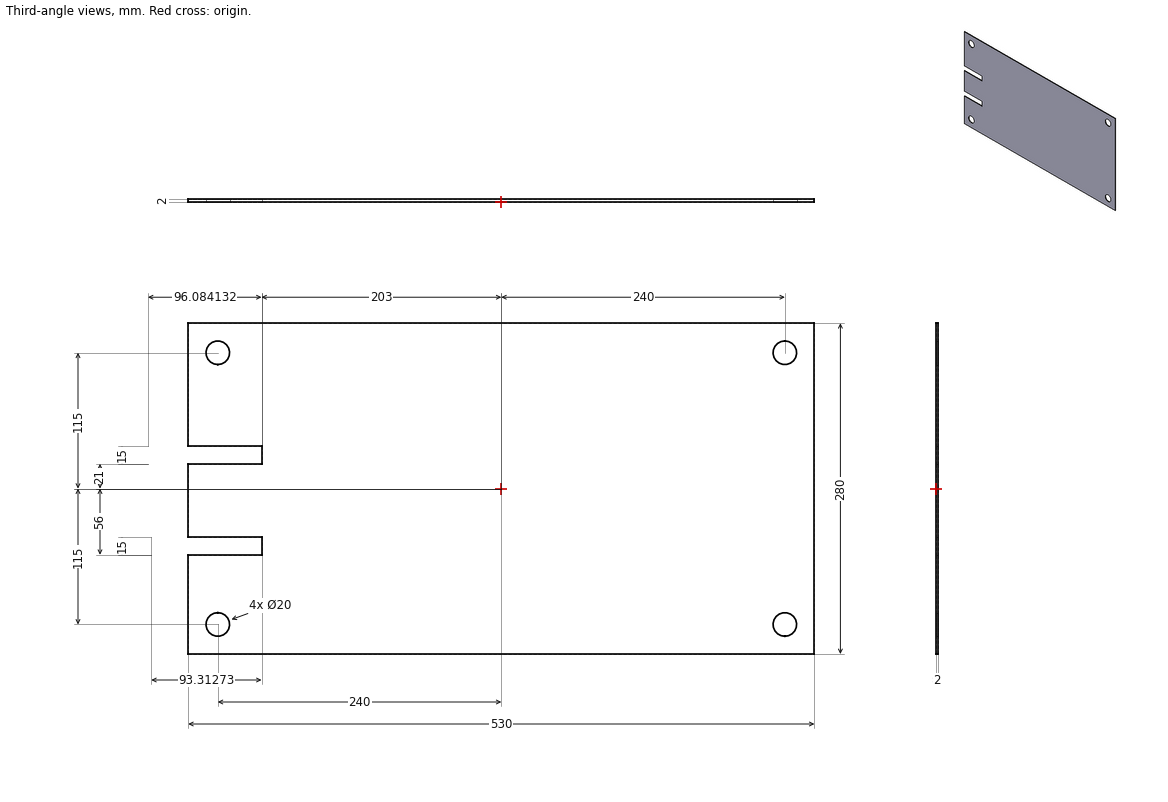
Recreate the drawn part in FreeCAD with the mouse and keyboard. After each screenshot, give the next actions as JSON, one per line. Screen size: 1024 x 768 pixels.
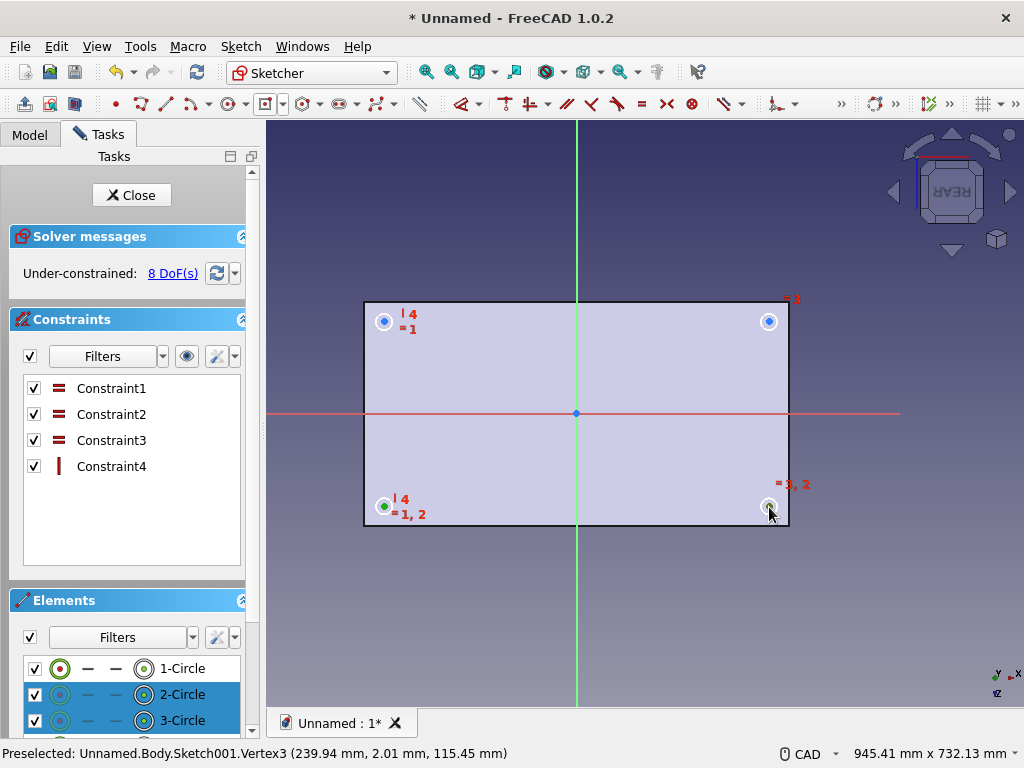
{"action": "left_click", "coordinate": [548, 104]}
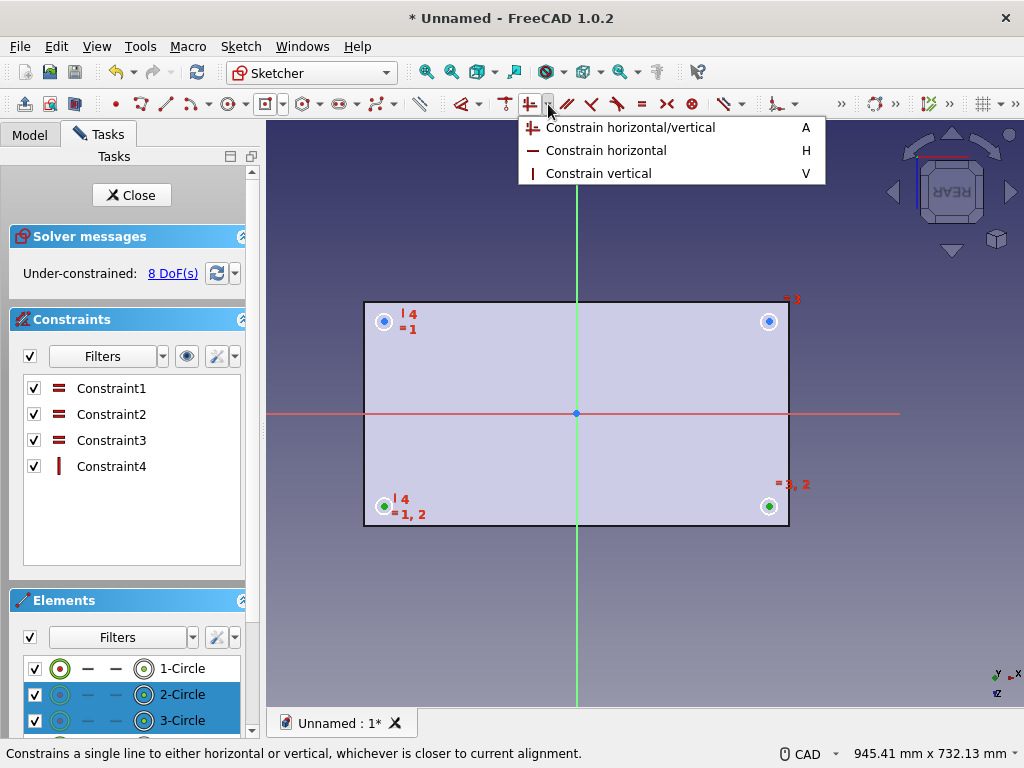
{"action": "left_click", "coordinate": [672, 150]}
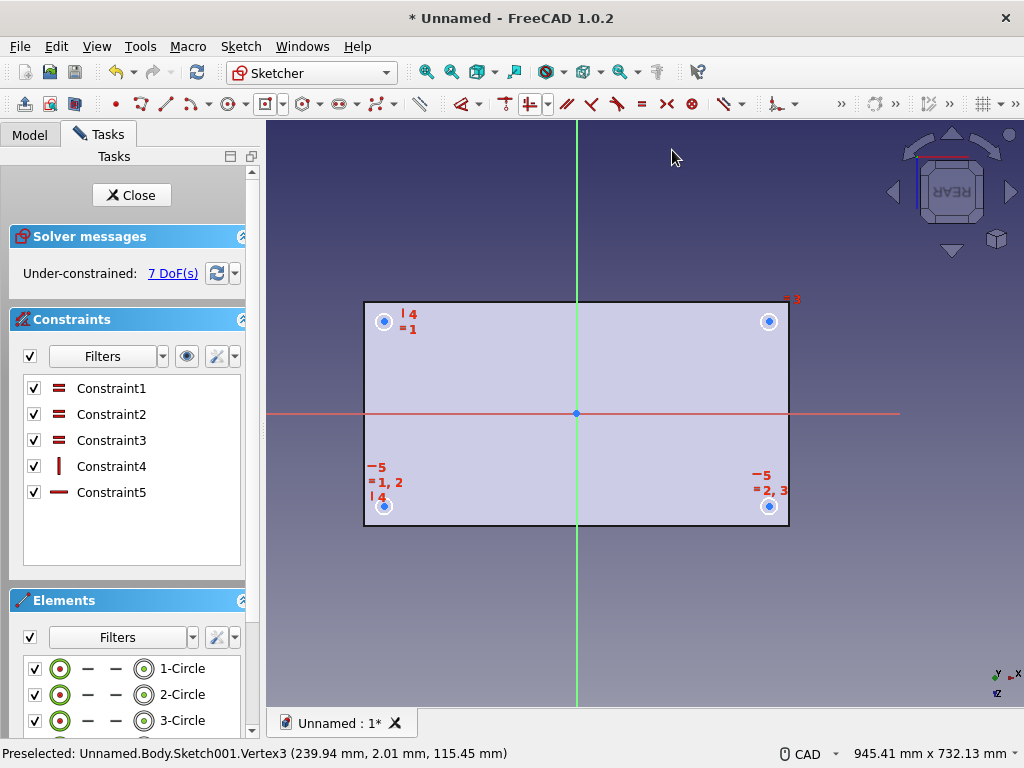
{"action": "left_click", "coordinate": [769, 506]}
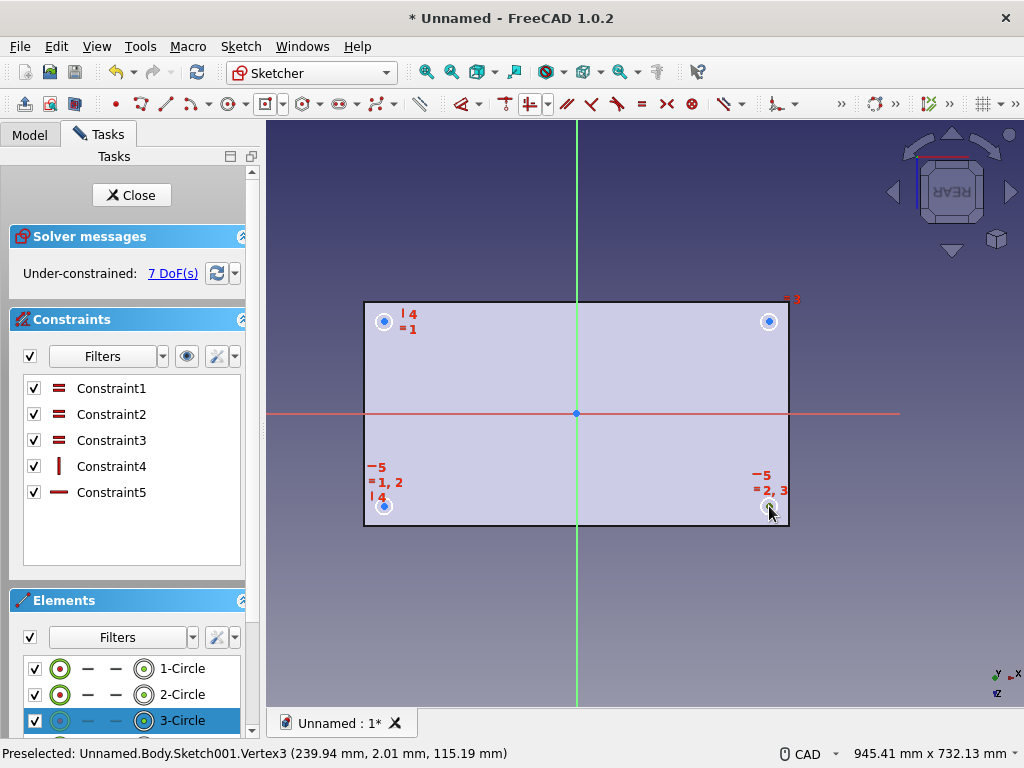
{"action": "left_click", "coordinate": [769, 322]}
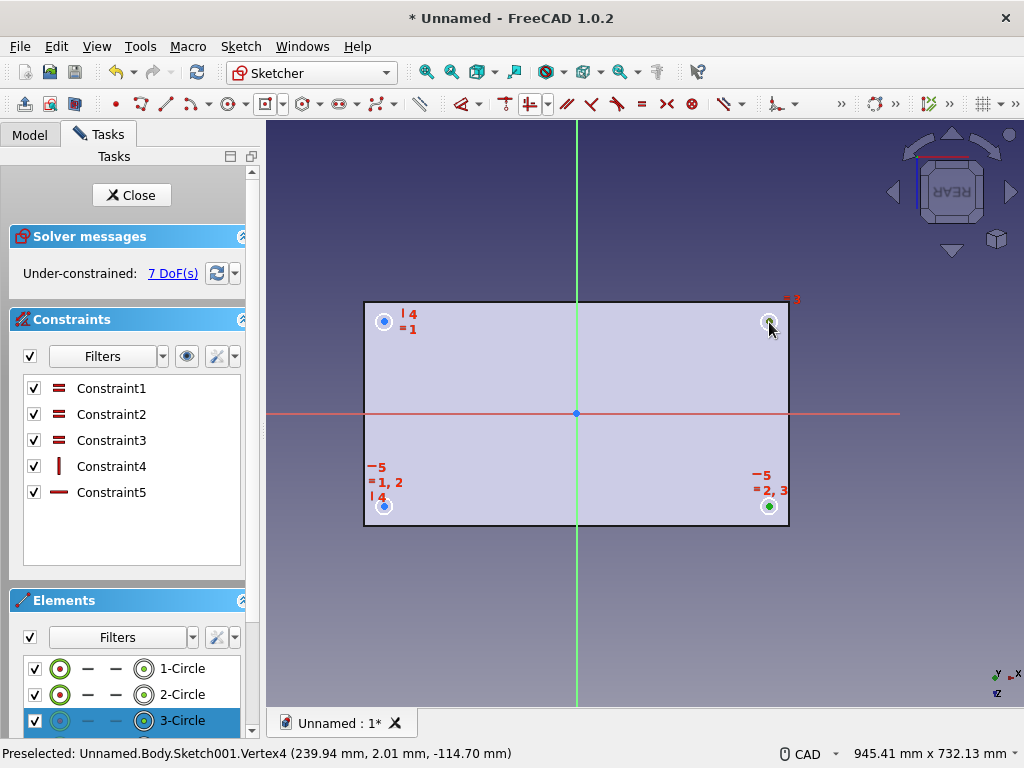
{"action": "left_click", "coordinate": [548, 104]}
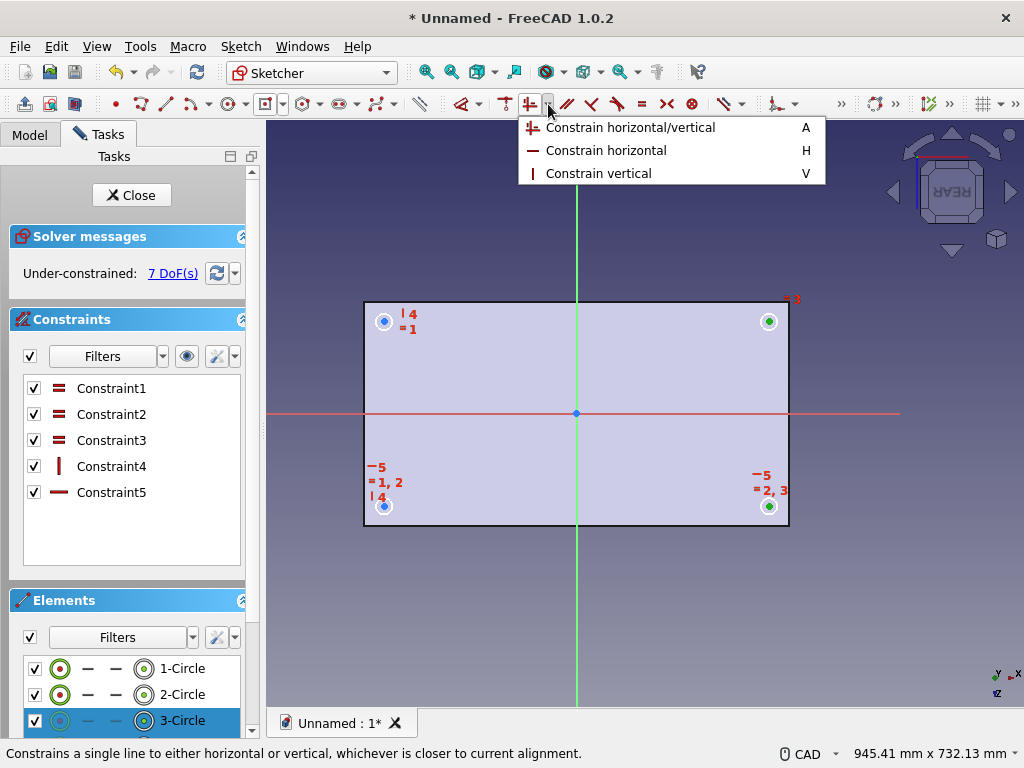
{"action": "left_click", "coordinate": [672, 174]}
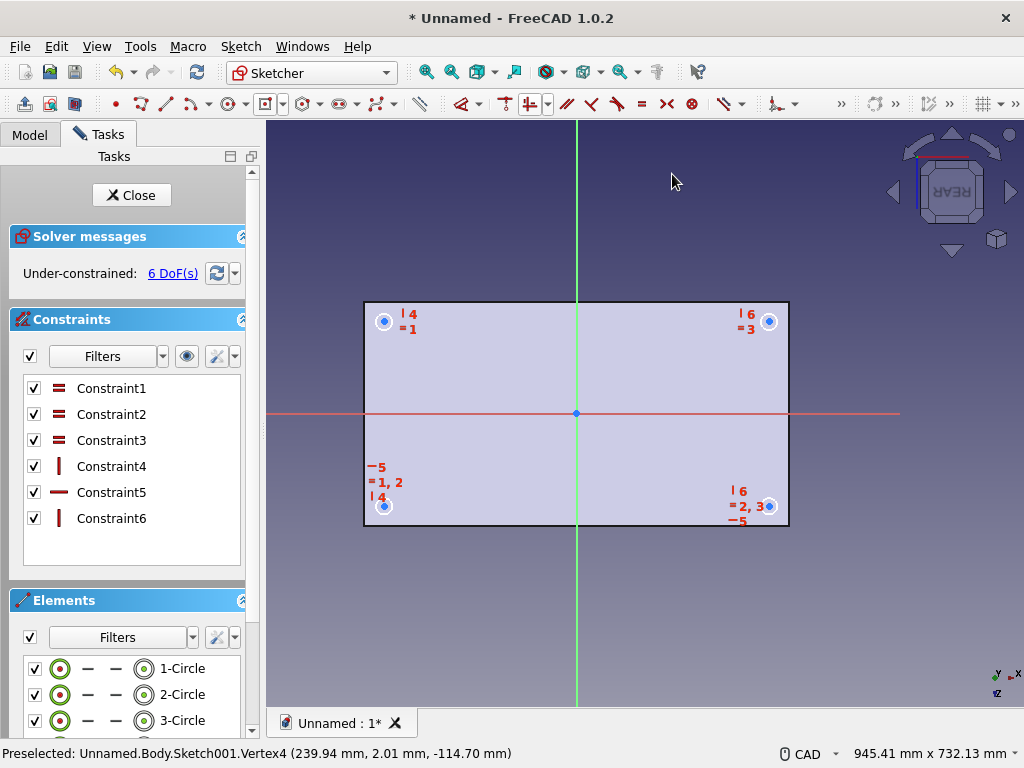
{"action": "left_click", "coordinate": [384, 322]}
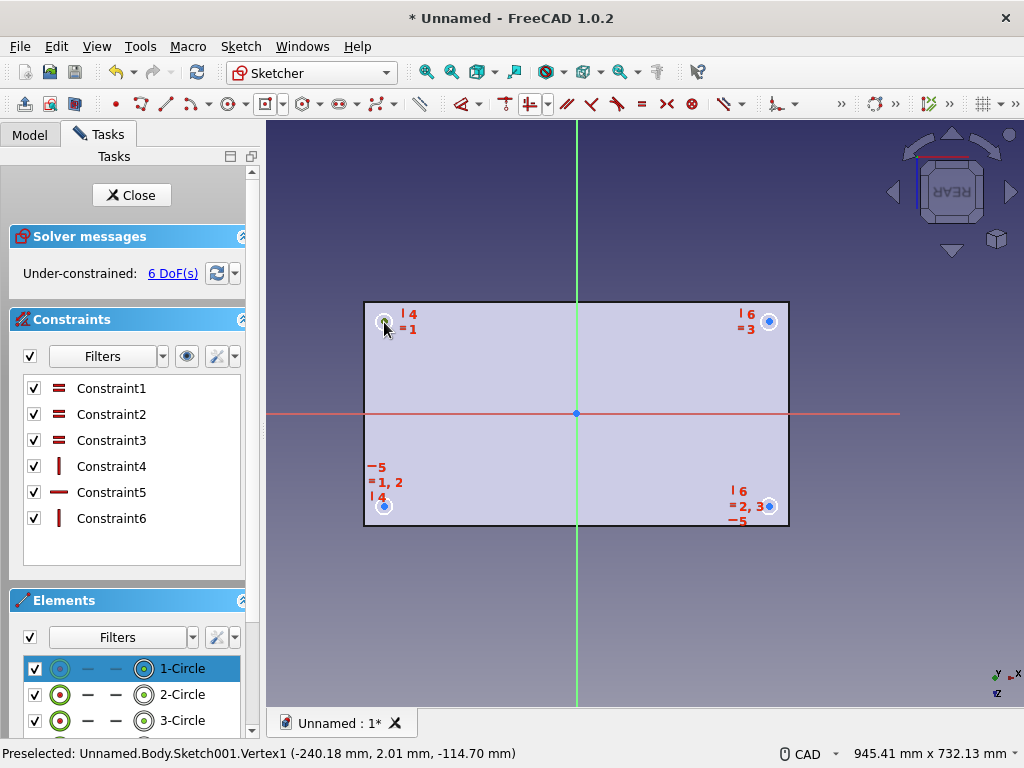
{"action": "left_click", "coordinate": [769, 322]}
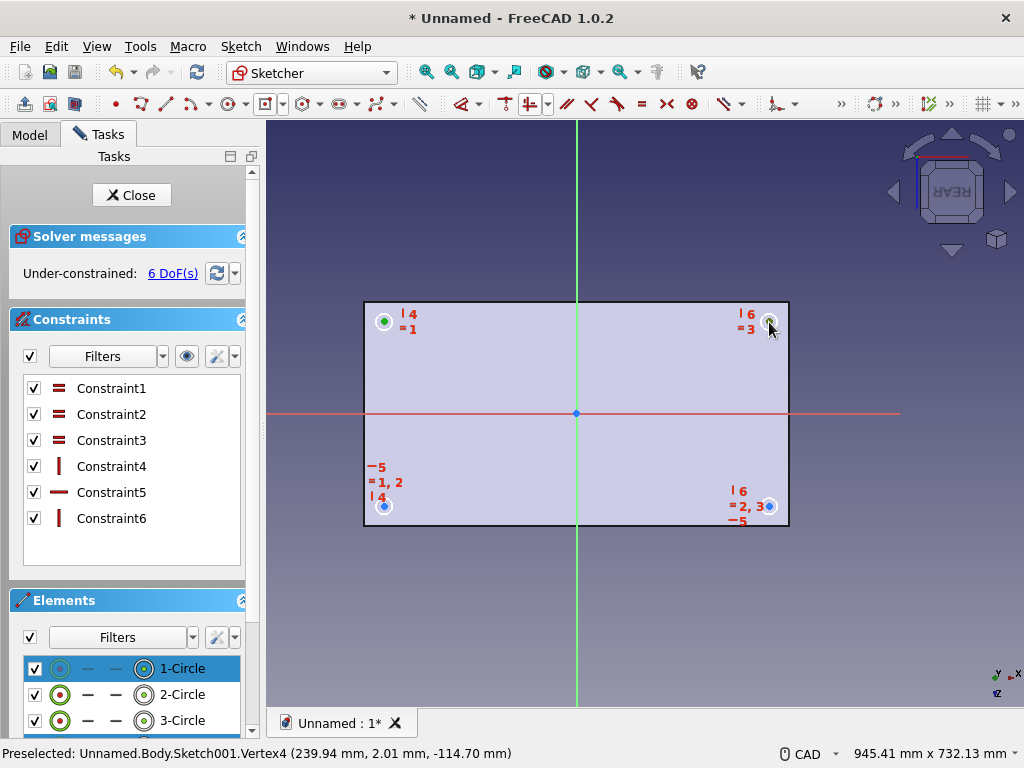
{"action": "left_click", "coordinate": [548, 104]}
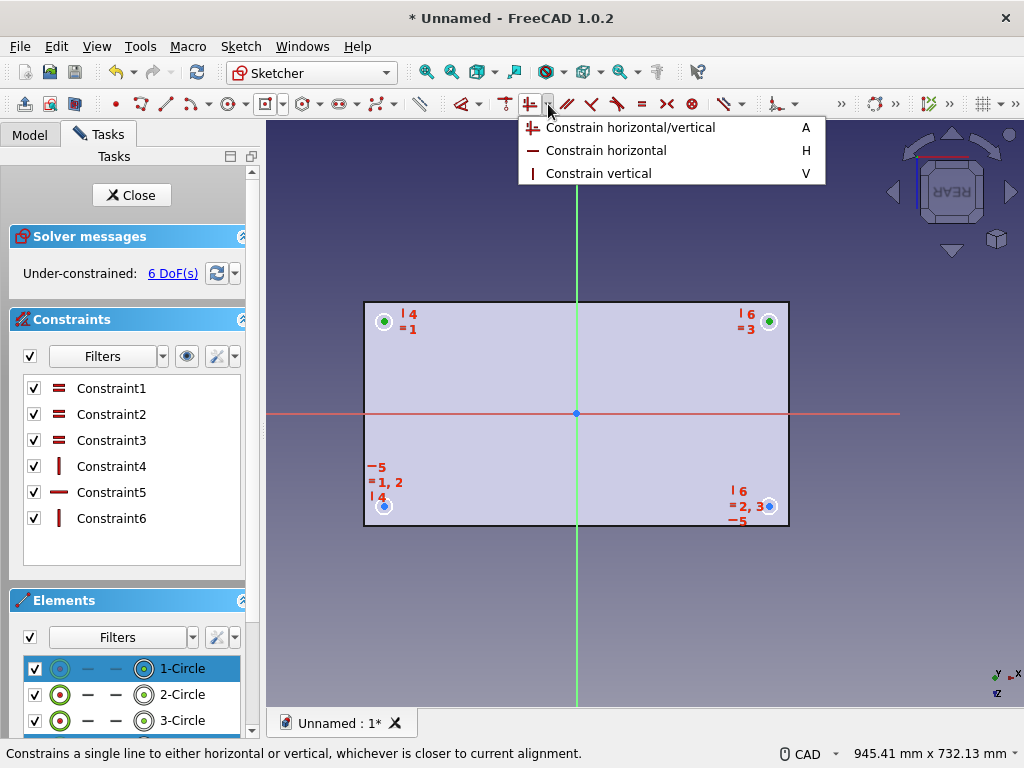
{"action": "left_click", "coordinate": [672, 150]}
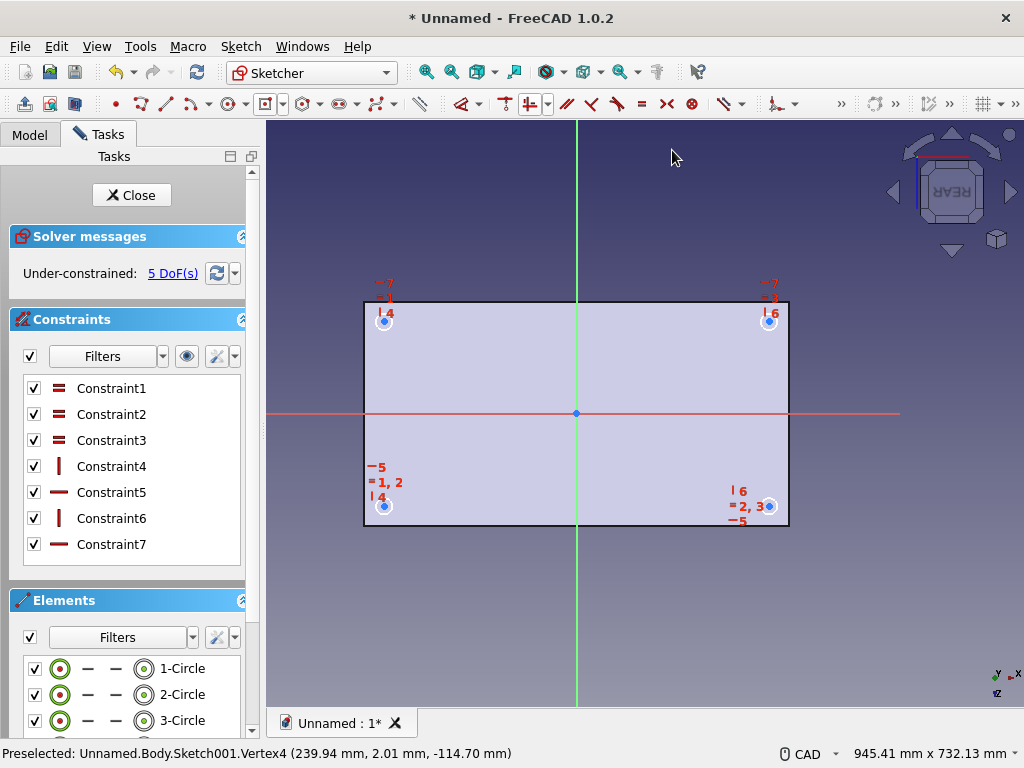
{"action": "left_click", "coordinate": [460, 104]}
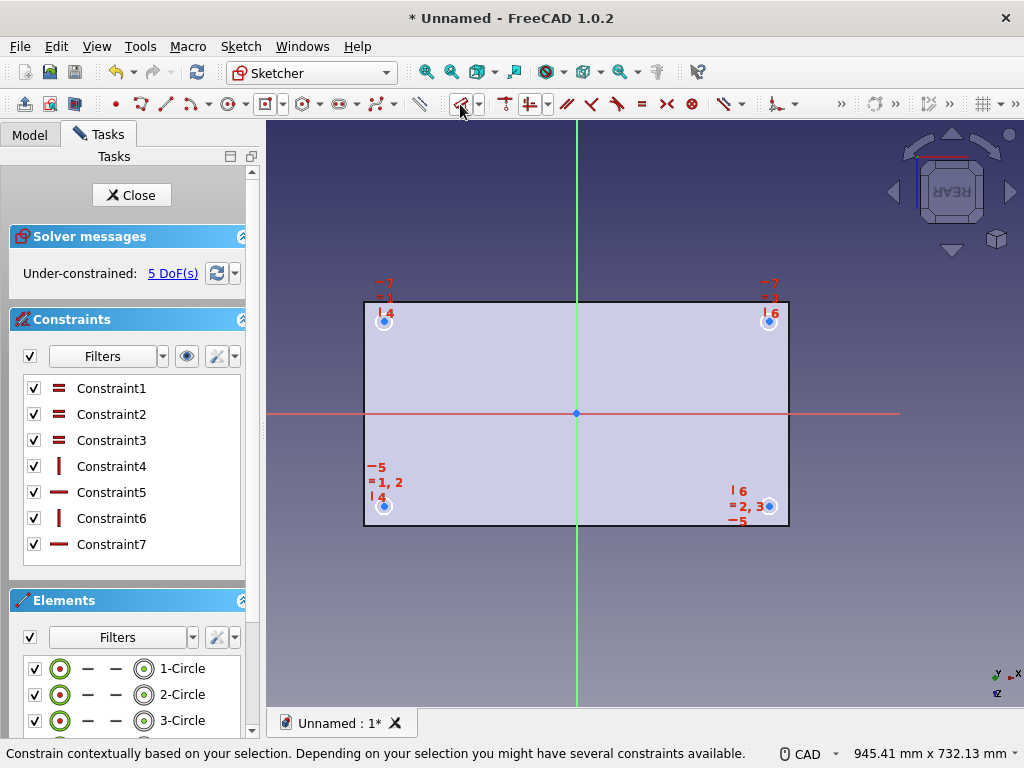
{"action": "scroll", "coordinate": [376, 322], "scroll_direction": "up", "scroll_amount": 5}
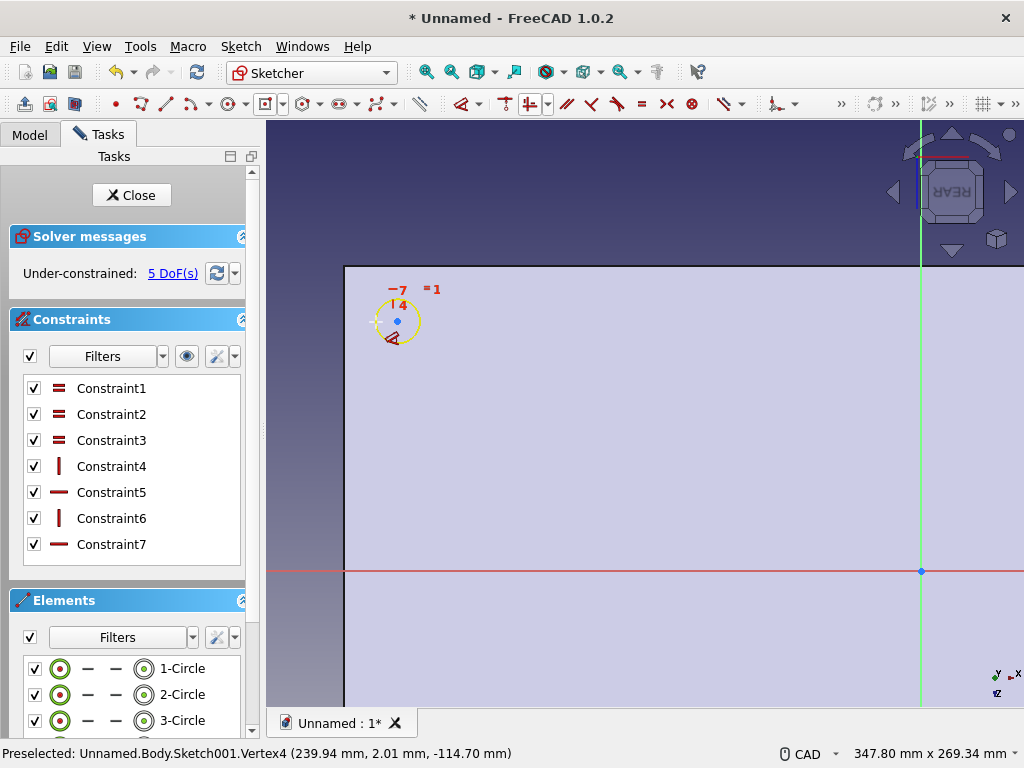
{"action": "left_click", "coordinate": [376, 321]}
{"action": "left_click", "coordinate": [344, 320]}